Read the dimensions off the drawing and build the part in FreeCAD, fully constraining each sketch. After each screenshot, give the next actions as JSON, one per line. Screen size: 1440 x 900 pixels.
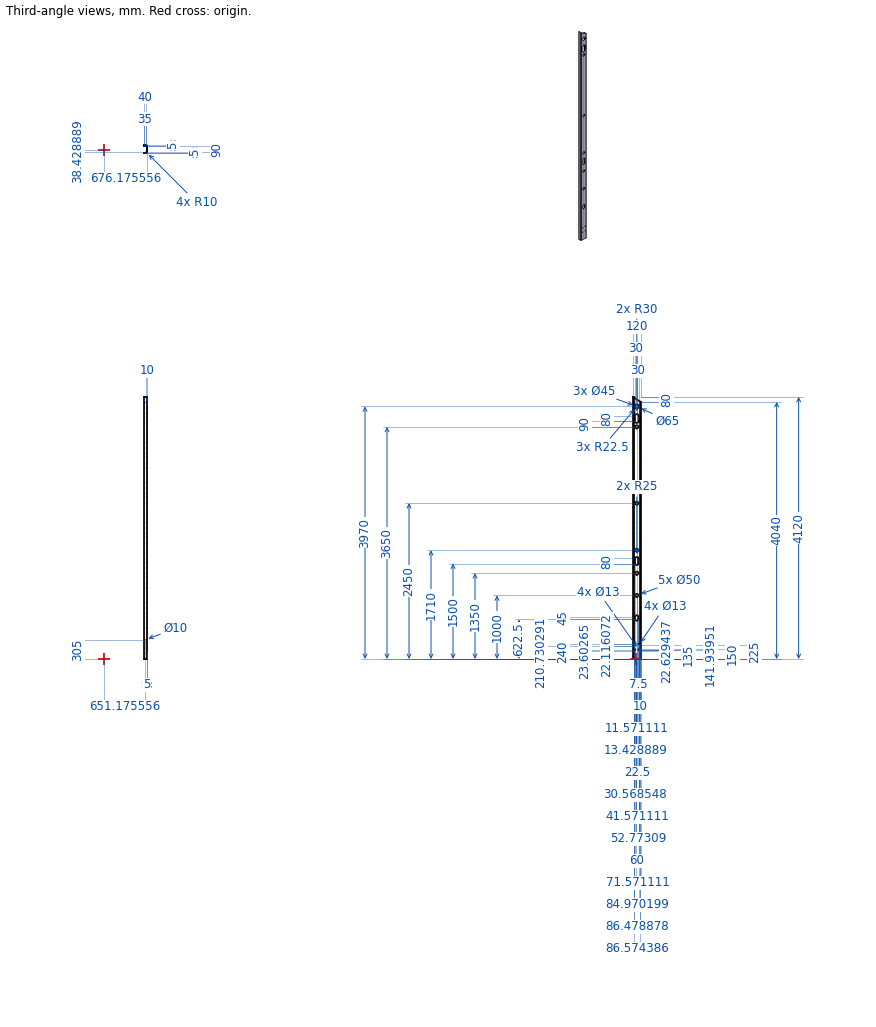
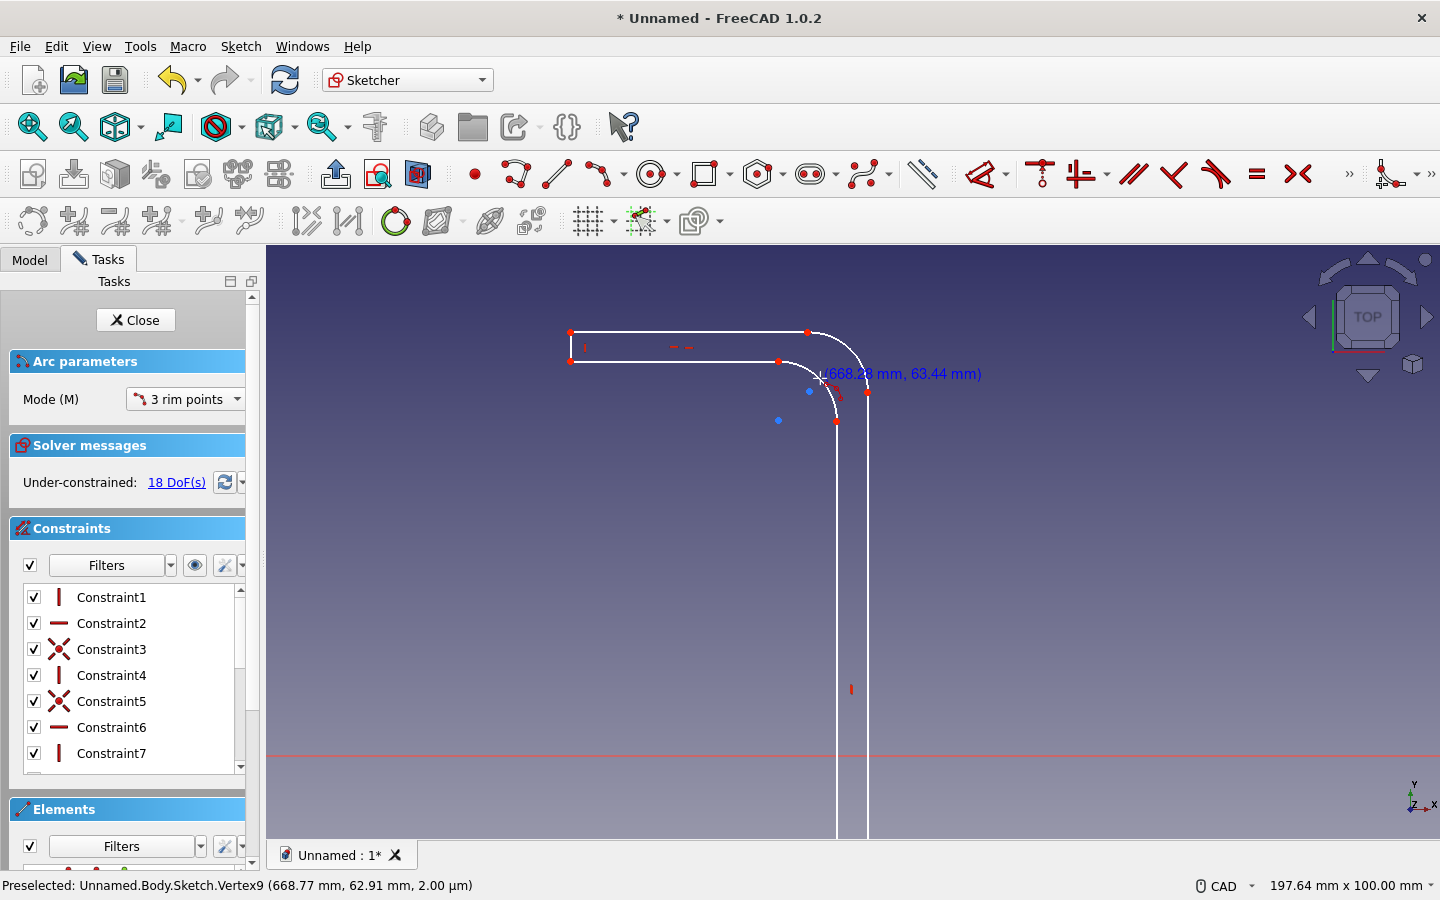
{"action": "scroll", "coordinate": [865, 366], "scroll_direction": "down", "scroll_amount": 3}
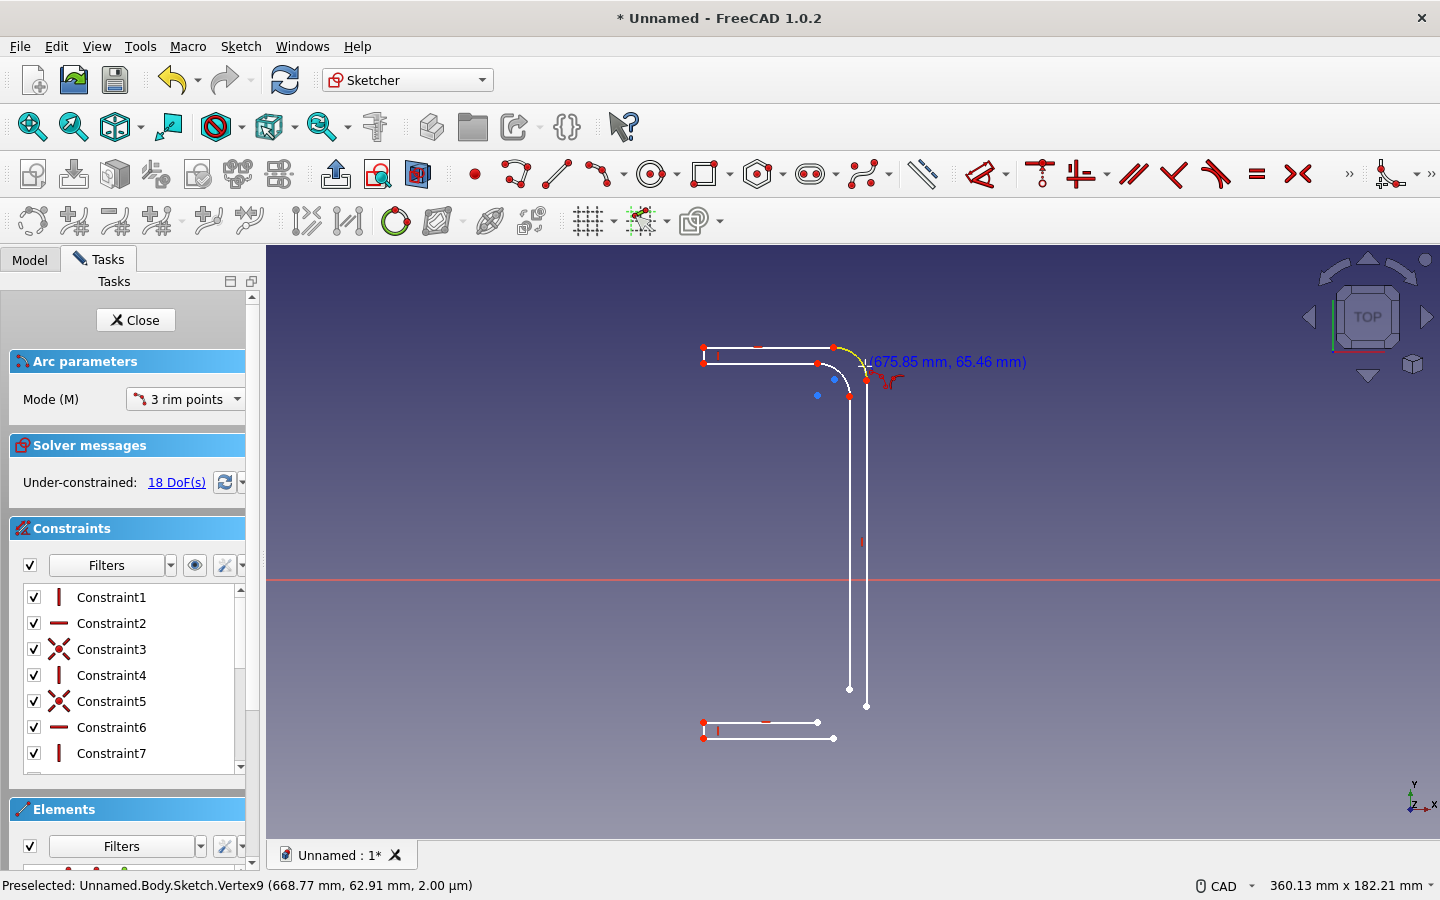
{"action": "left_click", "coordinate": [850, 690]}
{"action": "left_click", "coordinate": [818, 723]}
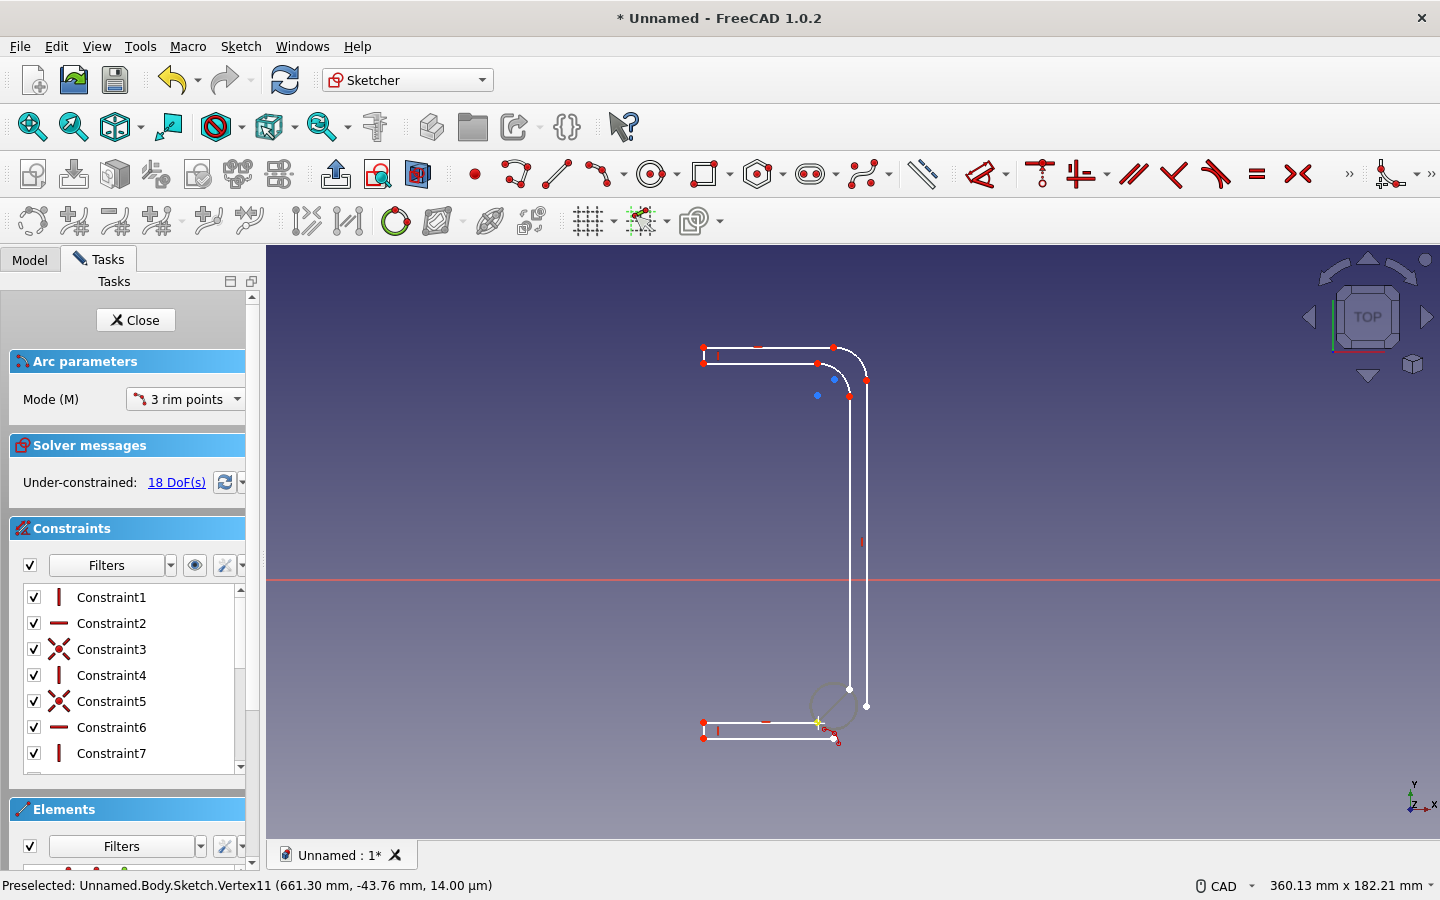
{"action": "scroll", "coordinate": [840, 712], "scroll_direction": "up", "scroll_amount": 3}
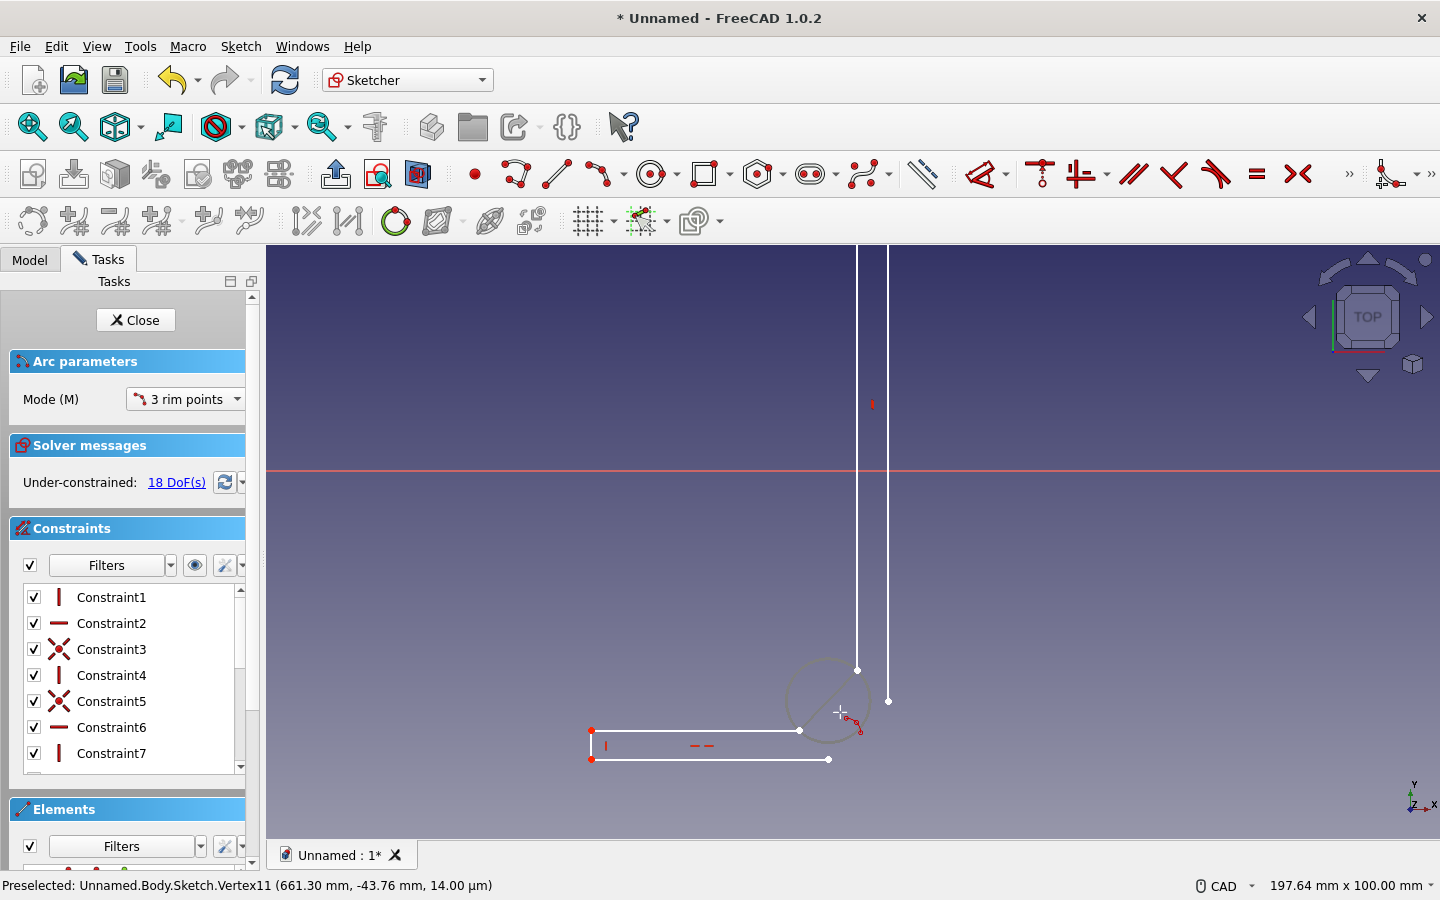
{"action": "left_click", "coordinate": [840, 711]}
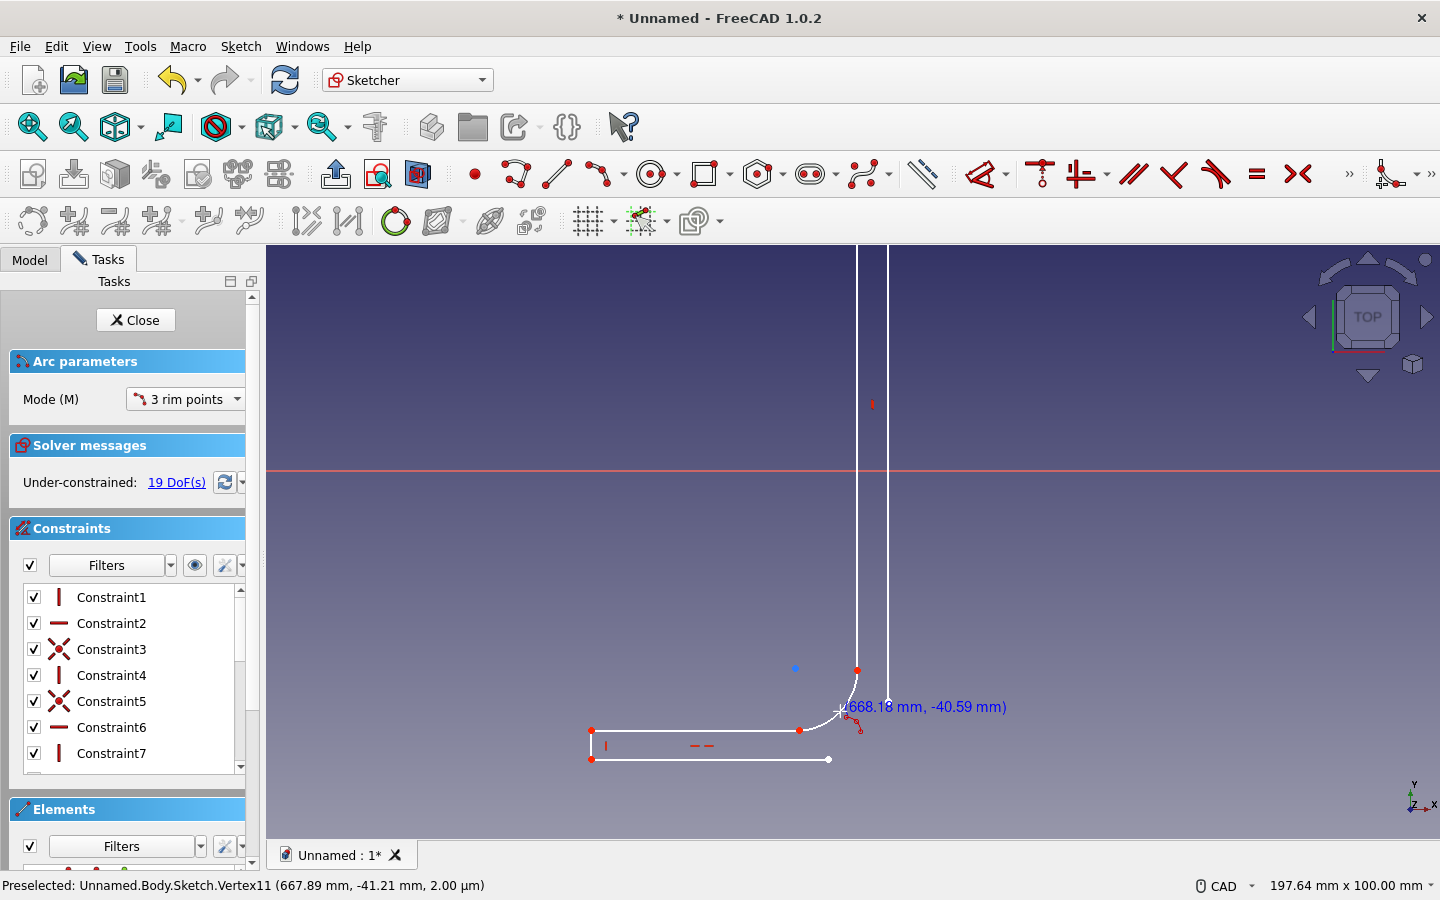
{"action": "left_click", "coordinate": [828, 760]}
{"action": "left_click", "coordinate": [888, 702]}
{"action": "left_click", "coordinate": [870, 741]}
{"action": "key", "text": "Escape"}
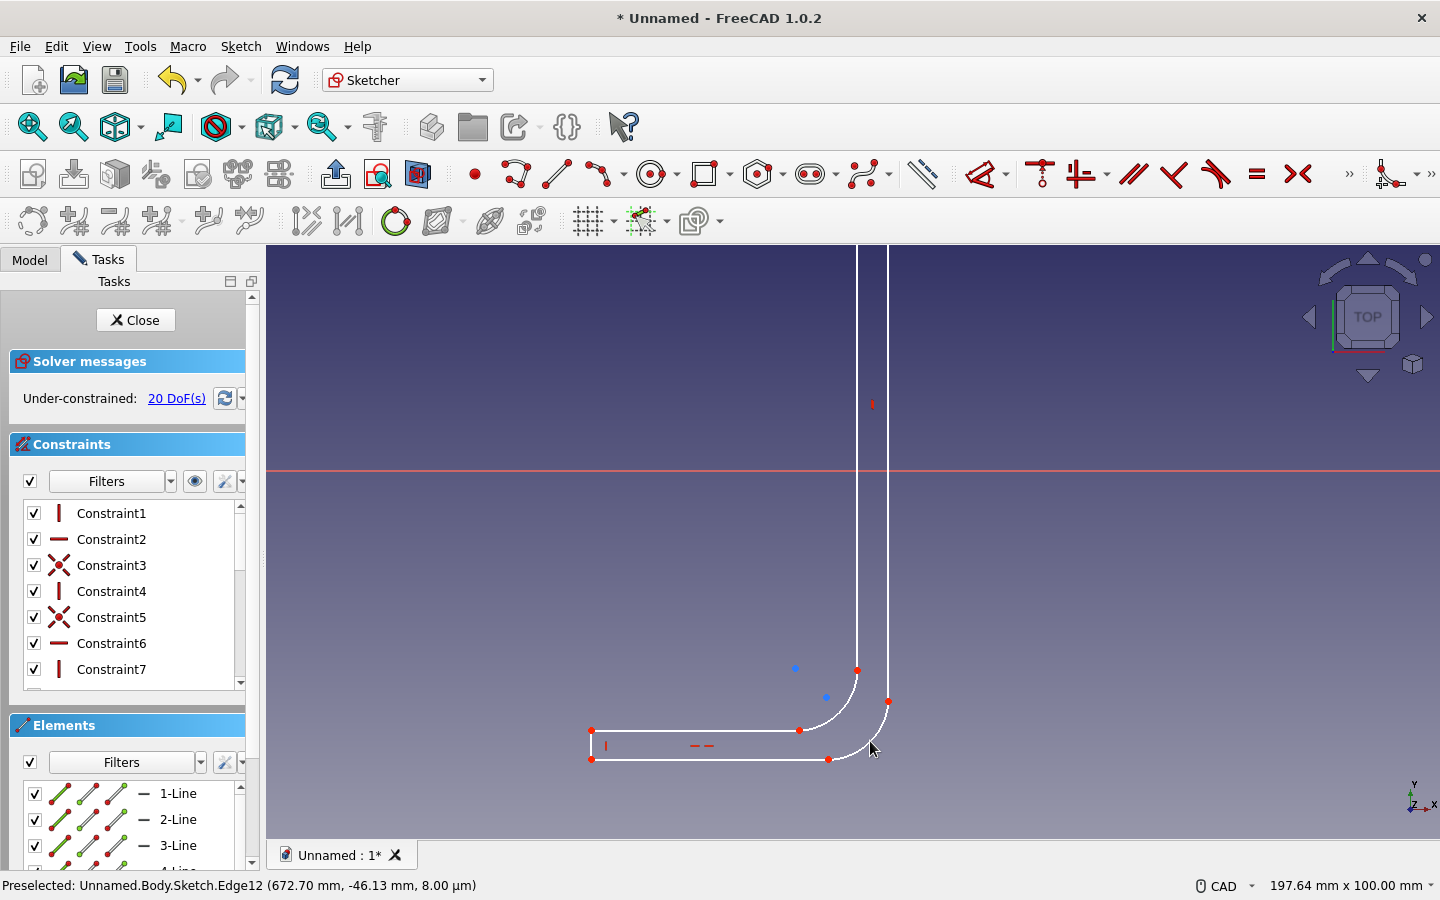
{"action": "left_click", "coordinate": [888, 523]}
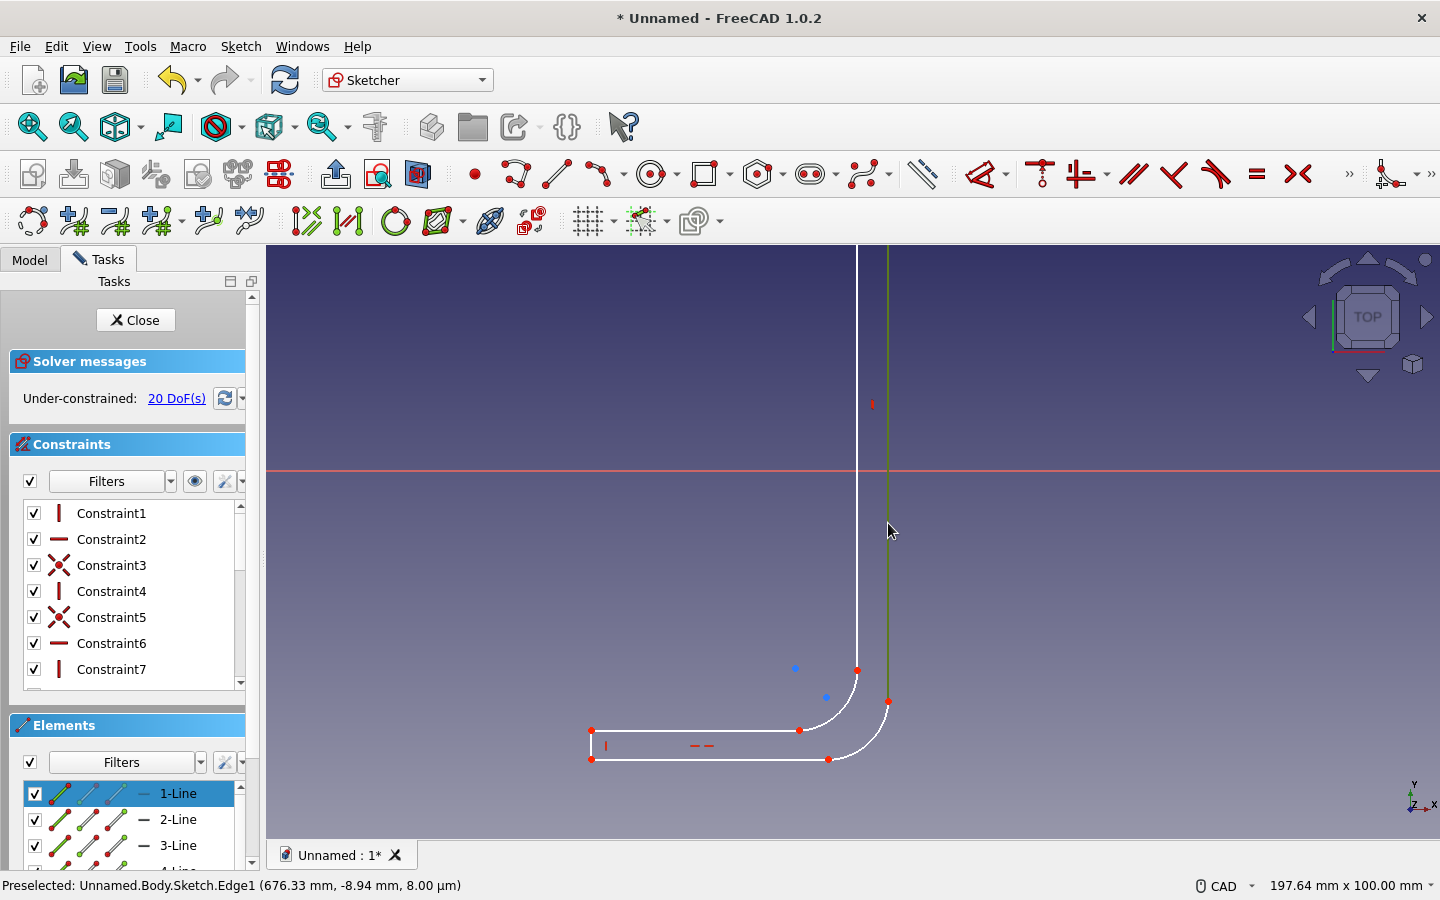
{"action": "scroll", "coordinate": [840, 712], "scroll_direction": "down", "scroll_amount": 3}